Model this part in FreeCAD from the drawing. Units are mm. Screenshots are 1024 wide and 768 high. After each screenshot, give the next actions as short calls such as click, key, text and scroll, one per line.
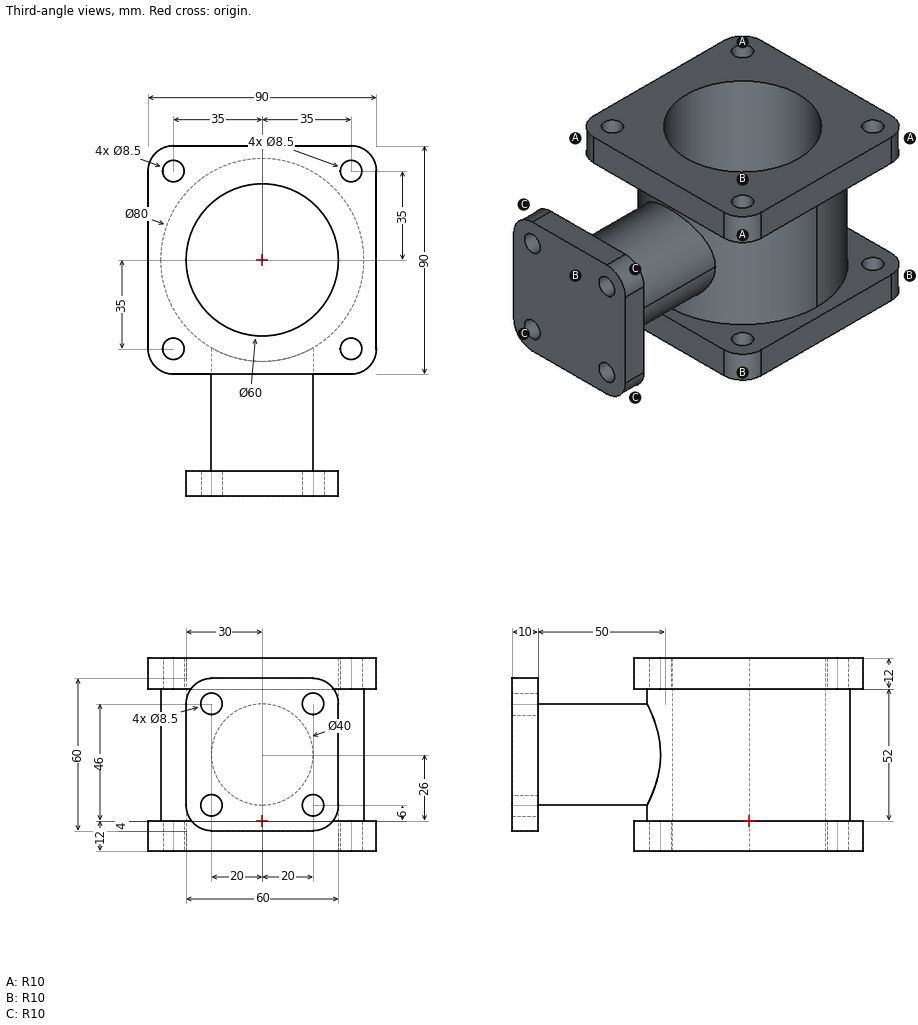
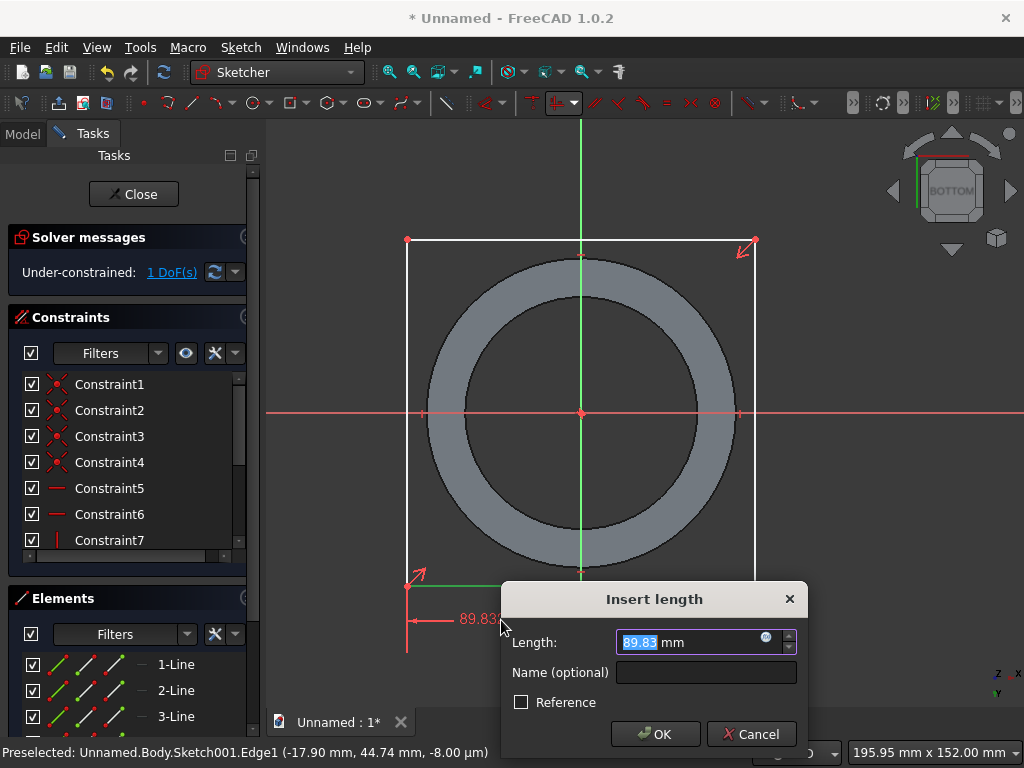
text(90)
key(Return)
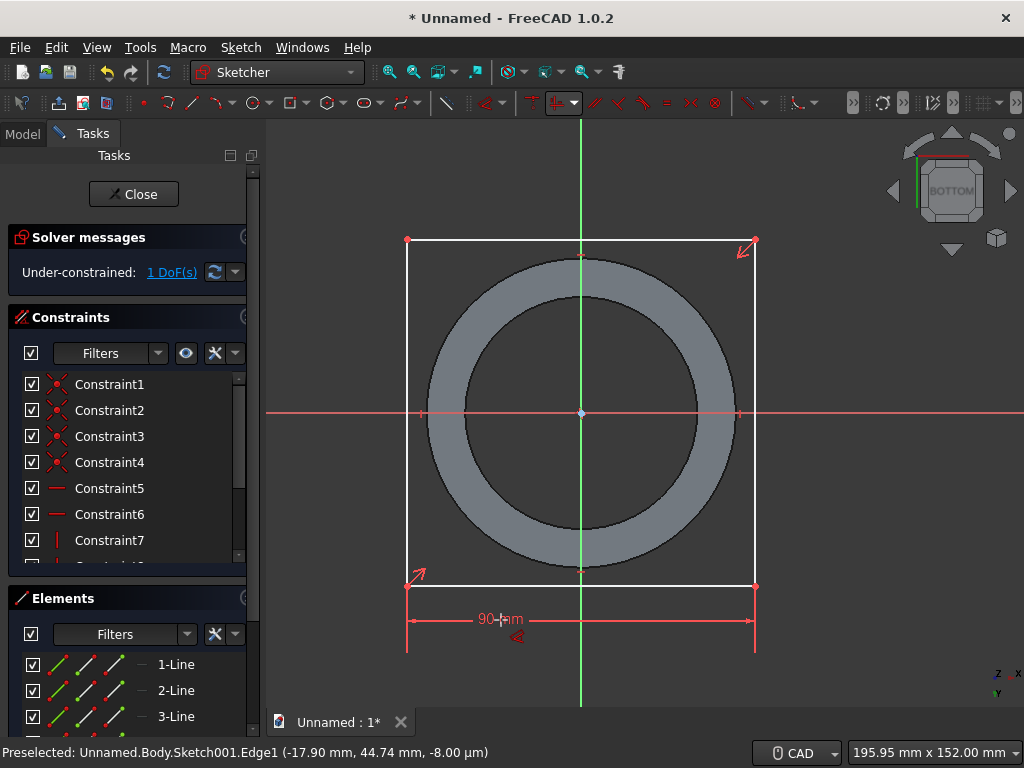
click(755, 482)
click(789, 333)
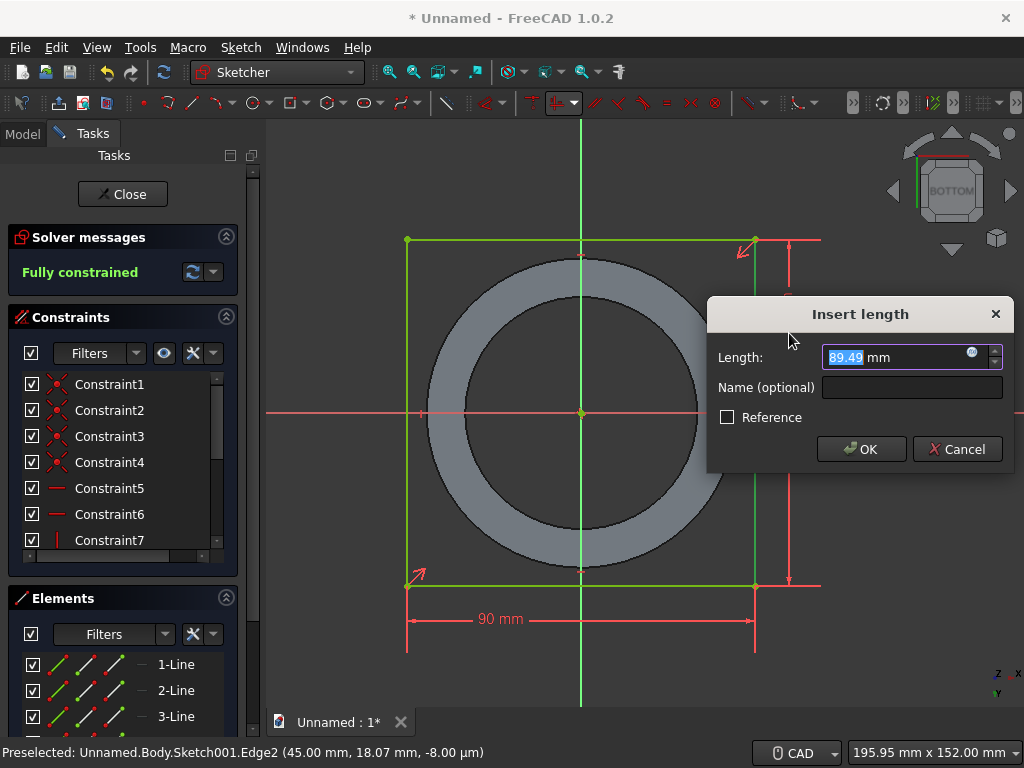
text(90)
key(Return)
key(Escape)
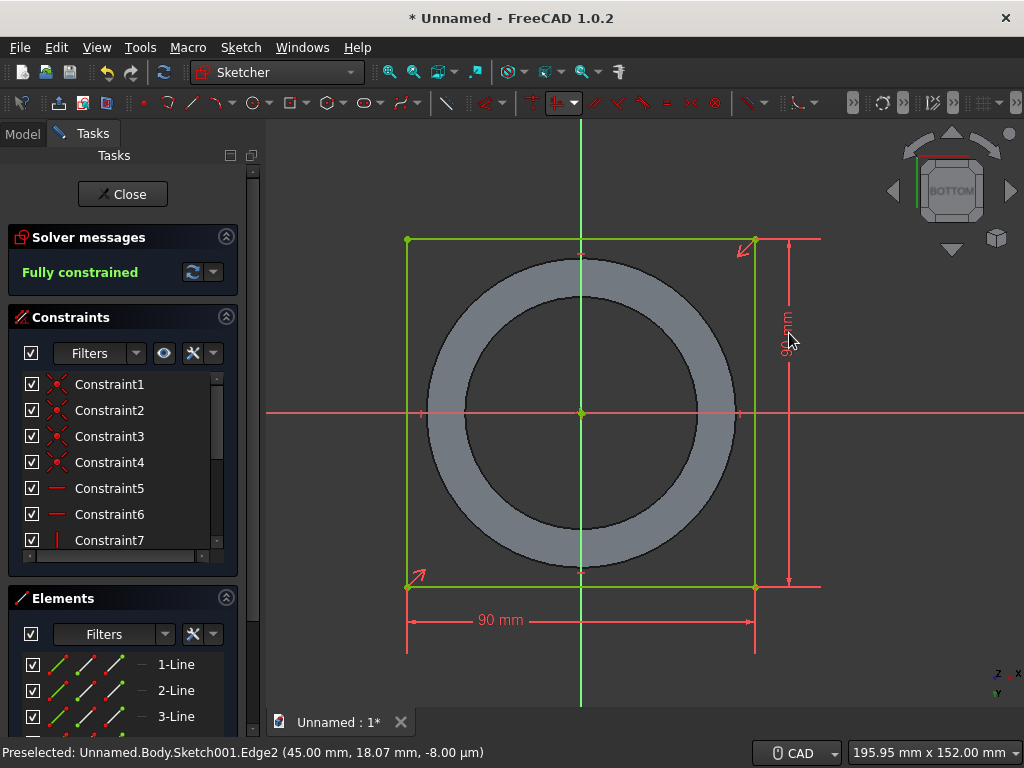
click(123, 194)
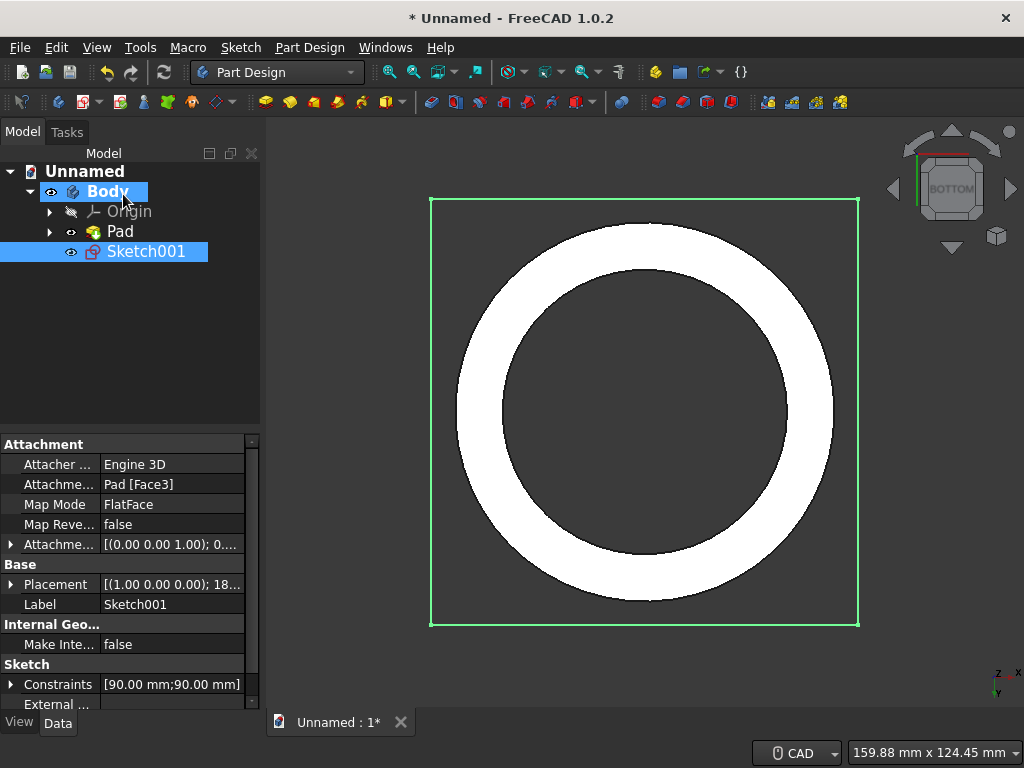
click(266, 102)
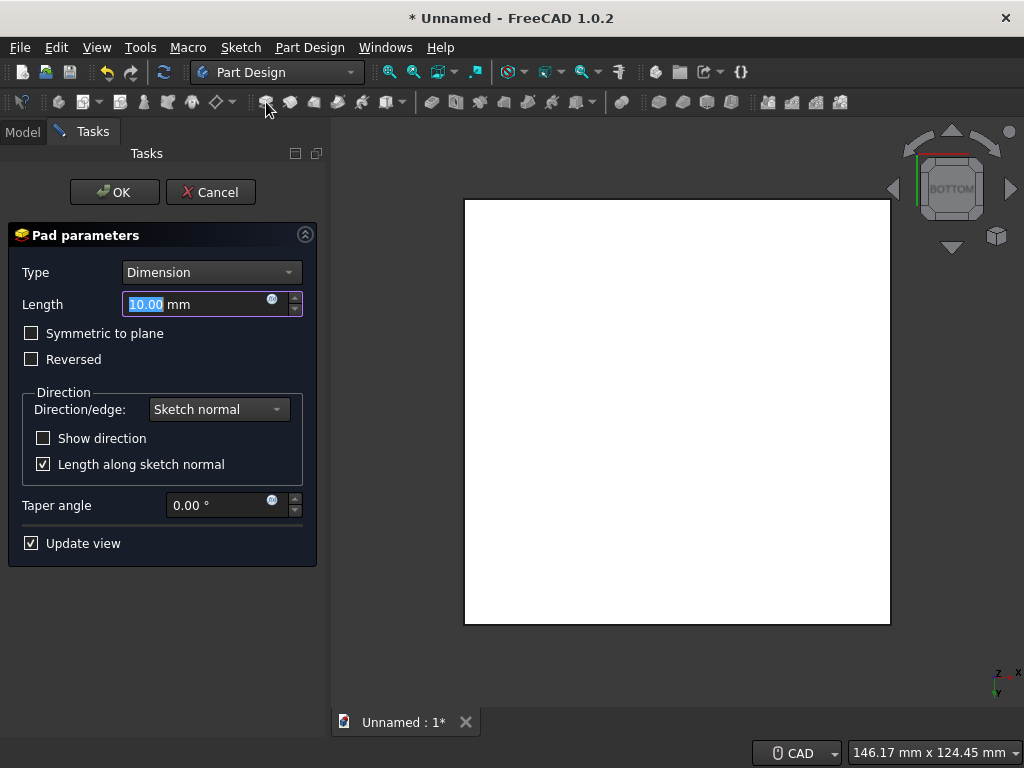
text(12)
key(Tab)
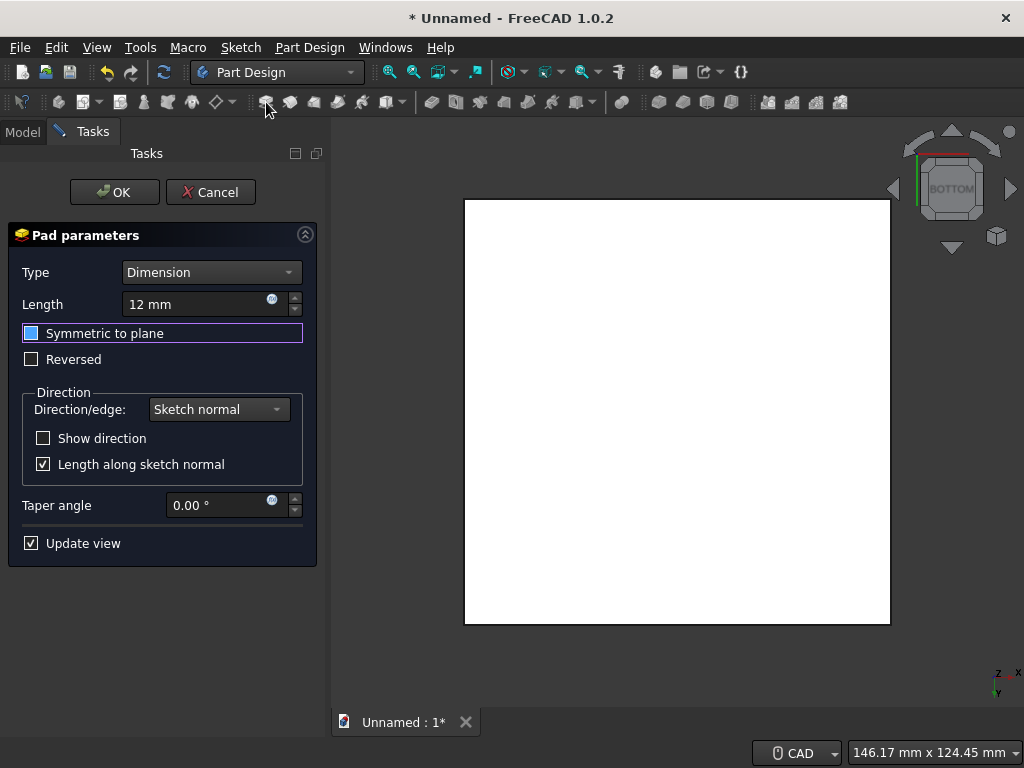
click(115, 192)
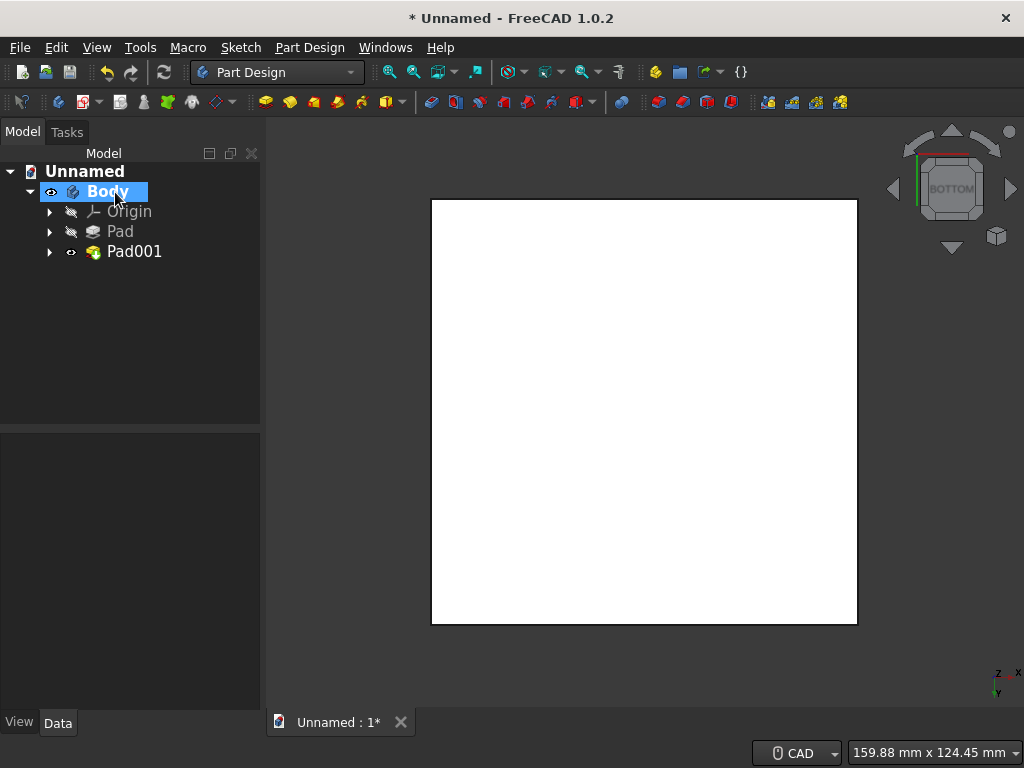
key(0)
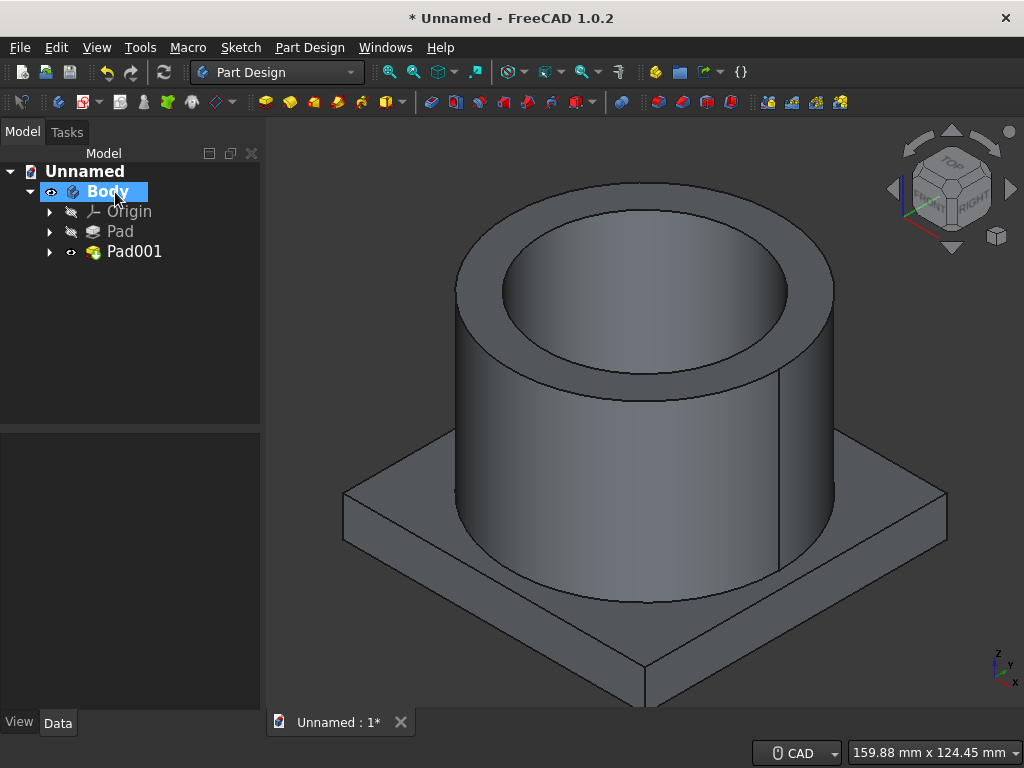
click(390, 72)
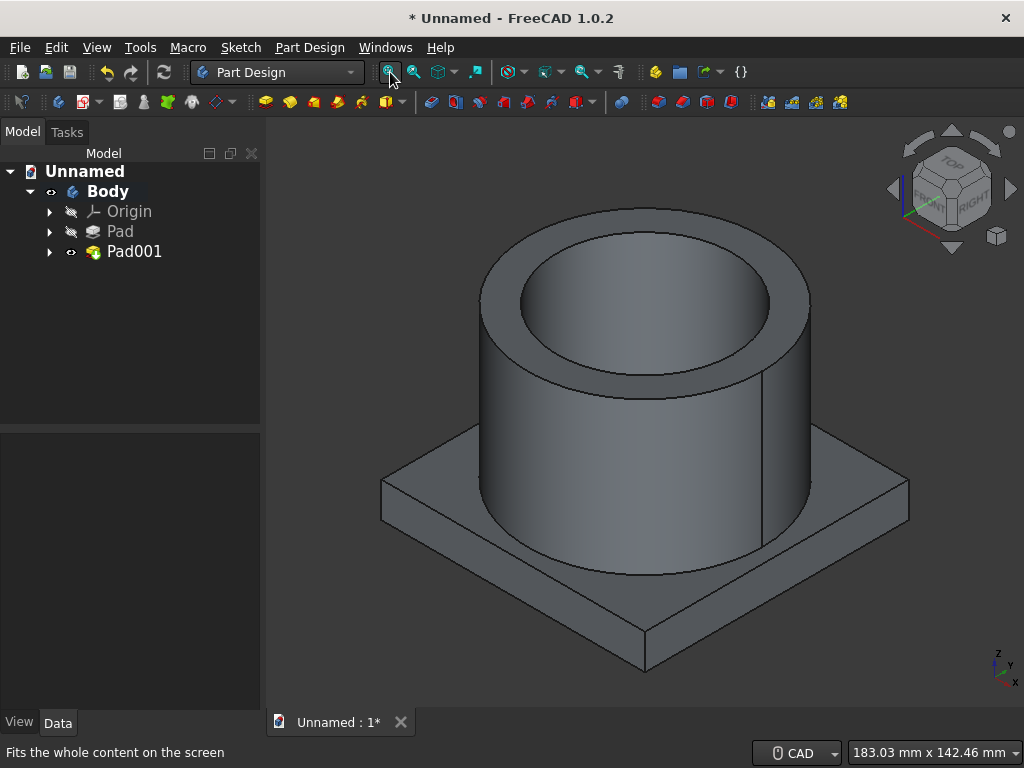
click(745, 361)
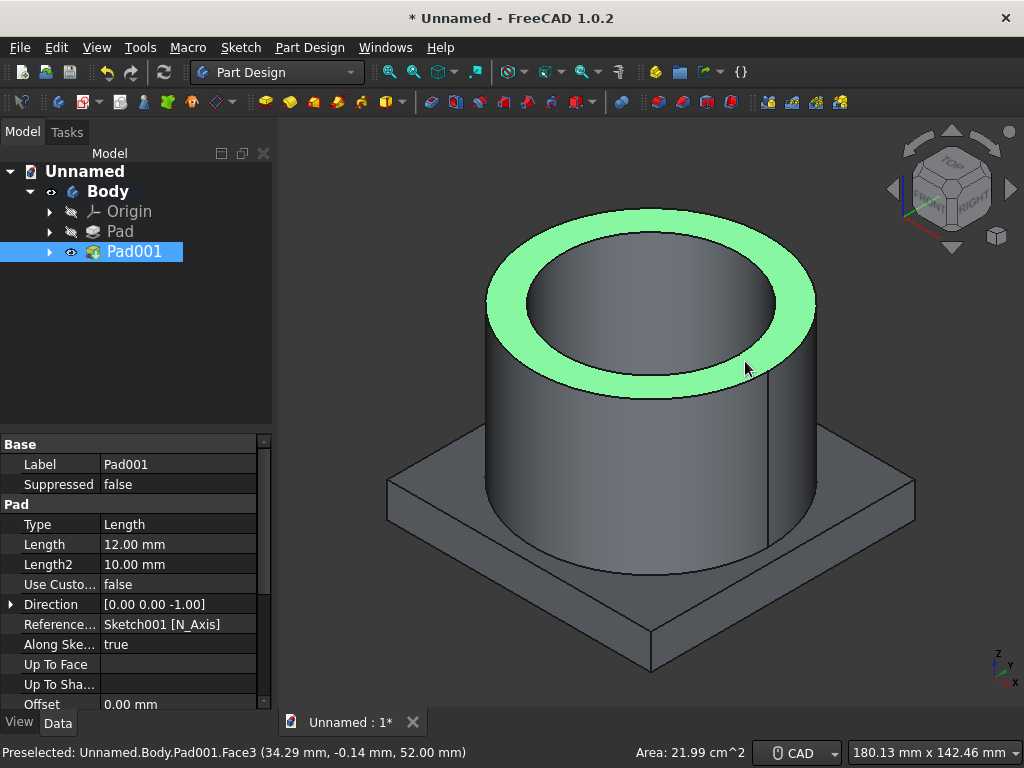
click(84, 102)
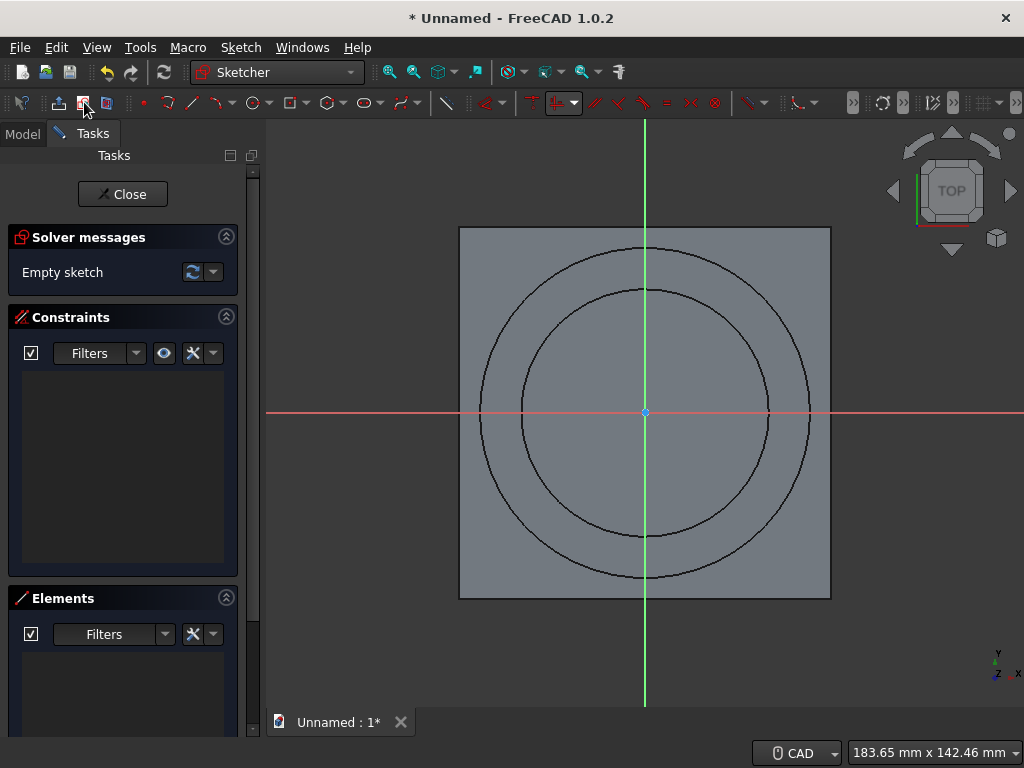
click(290, 104)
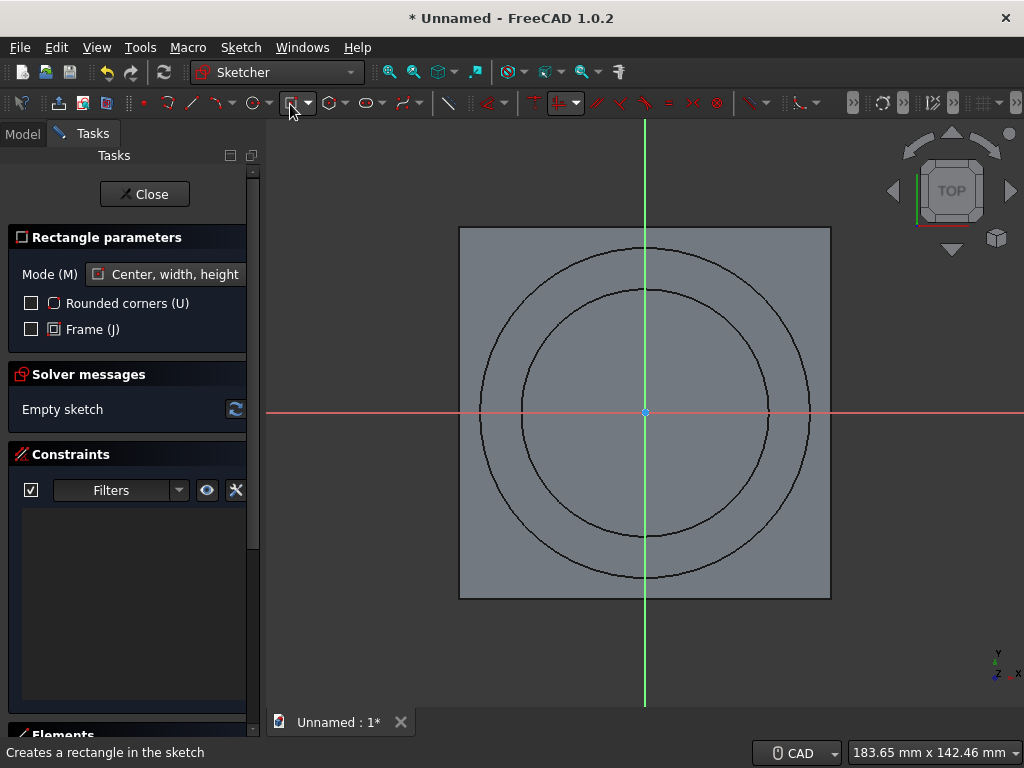
click(645, 413)
click(831, 227)
key(Escape)